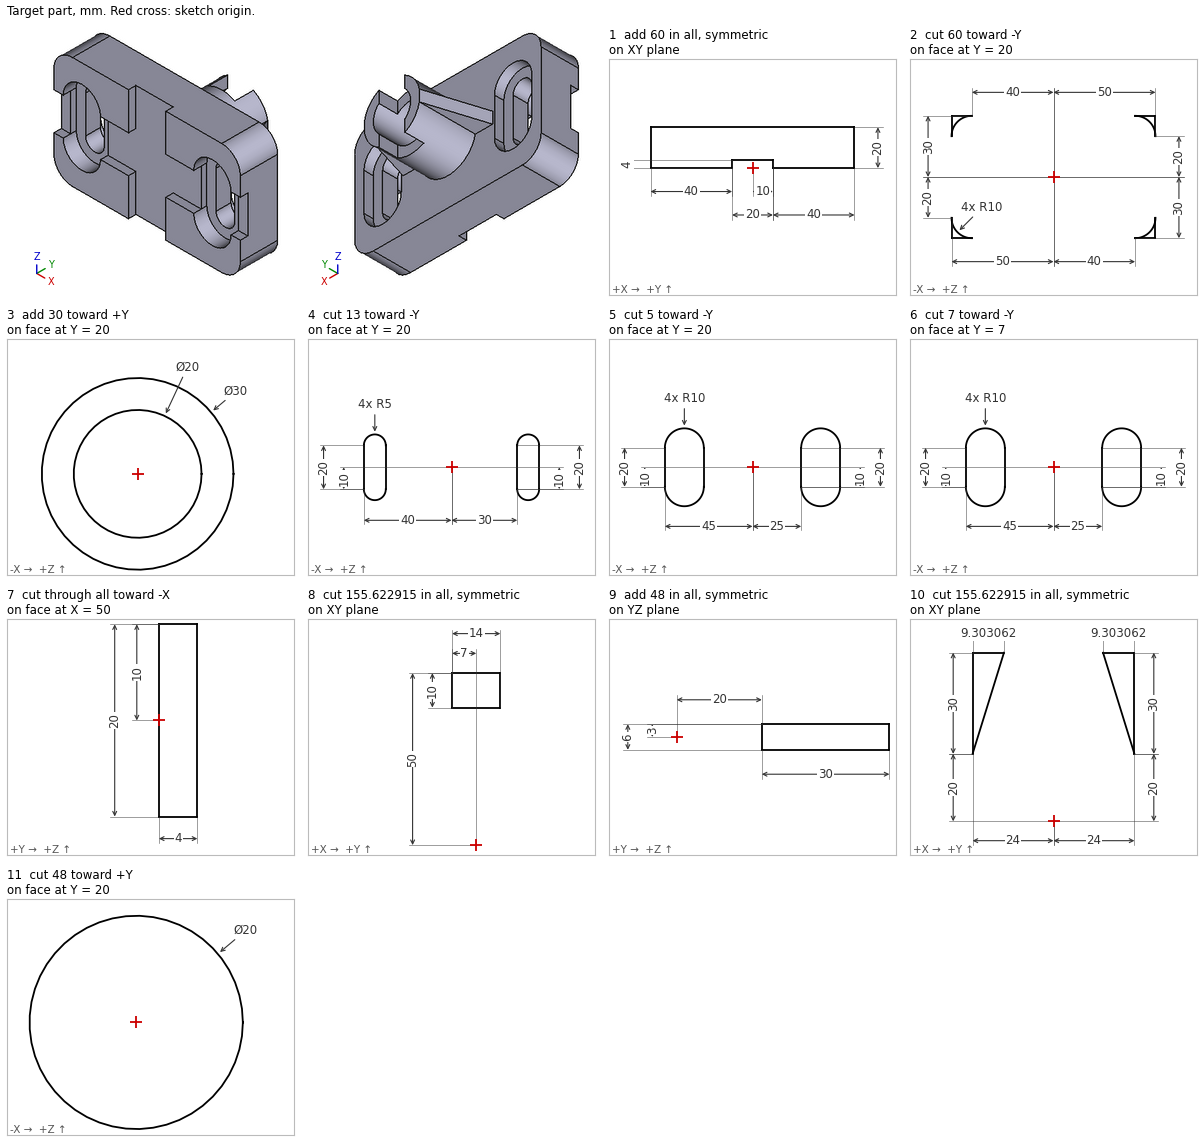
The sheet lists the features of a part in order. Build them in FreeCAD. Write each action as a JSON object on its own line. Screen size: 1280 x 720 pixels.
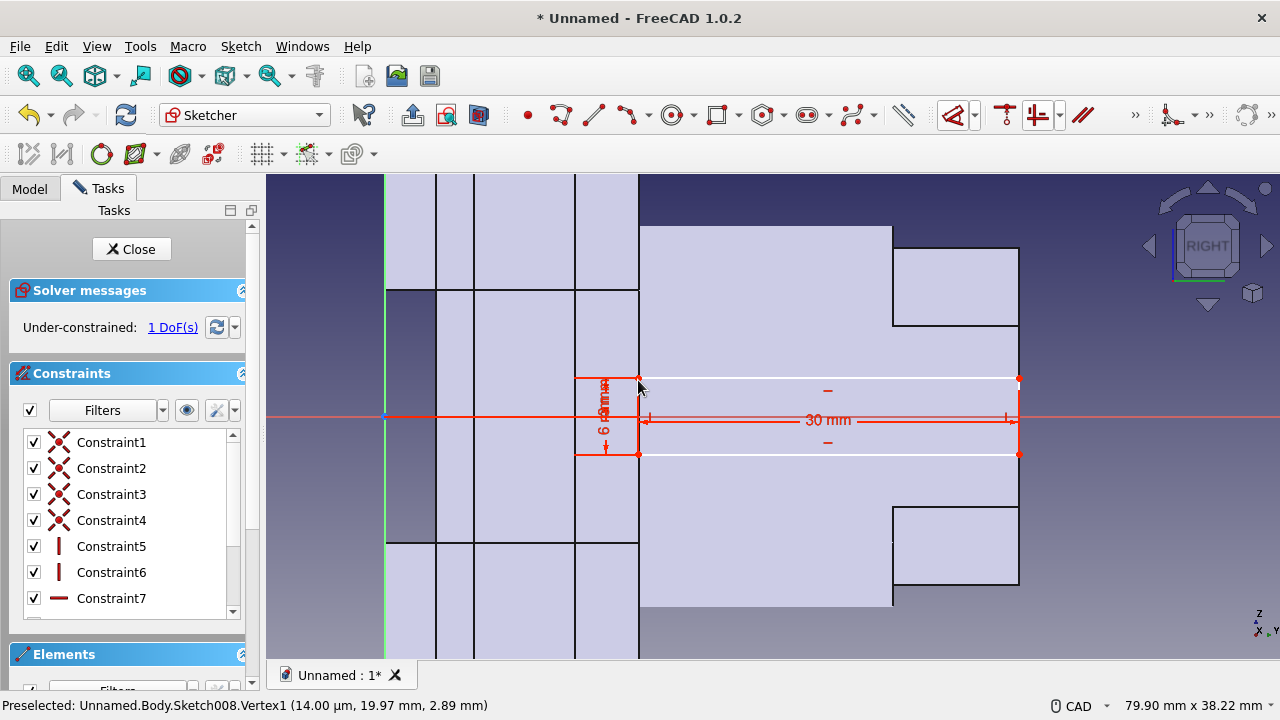
{"action": "left_click", "coordinate": [638, 378]}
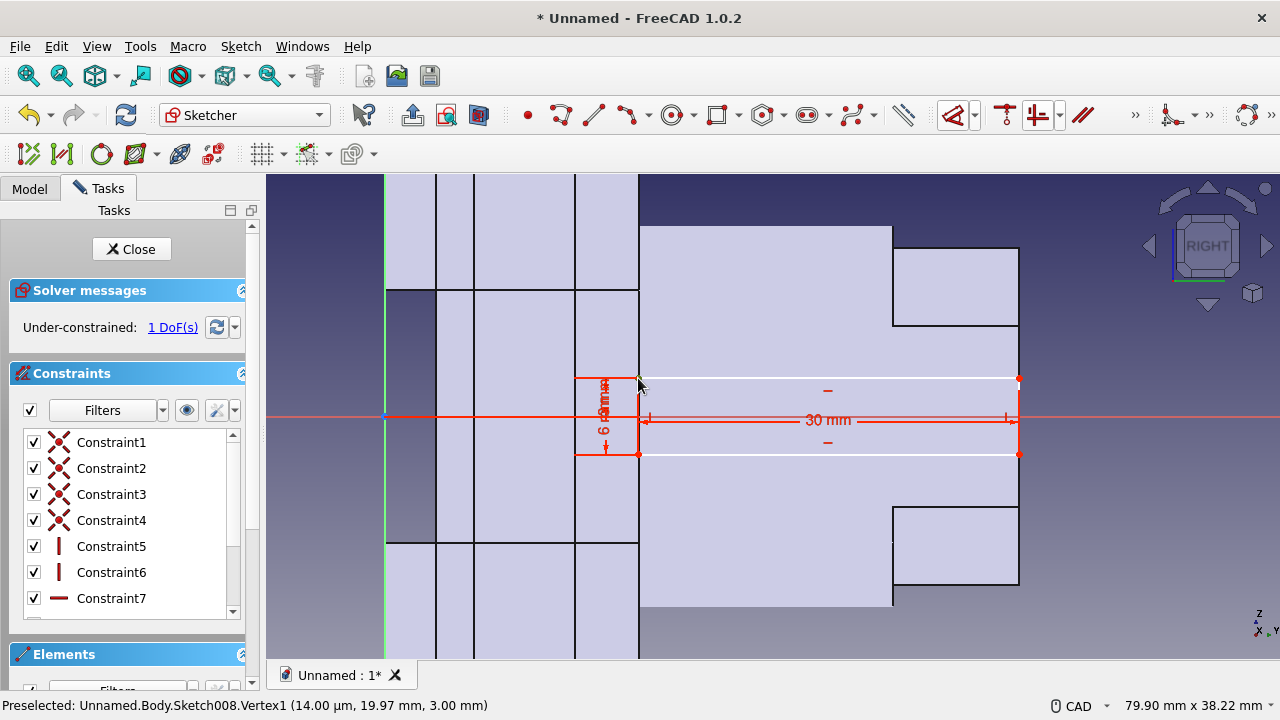
{"action": "key", "text": "l"}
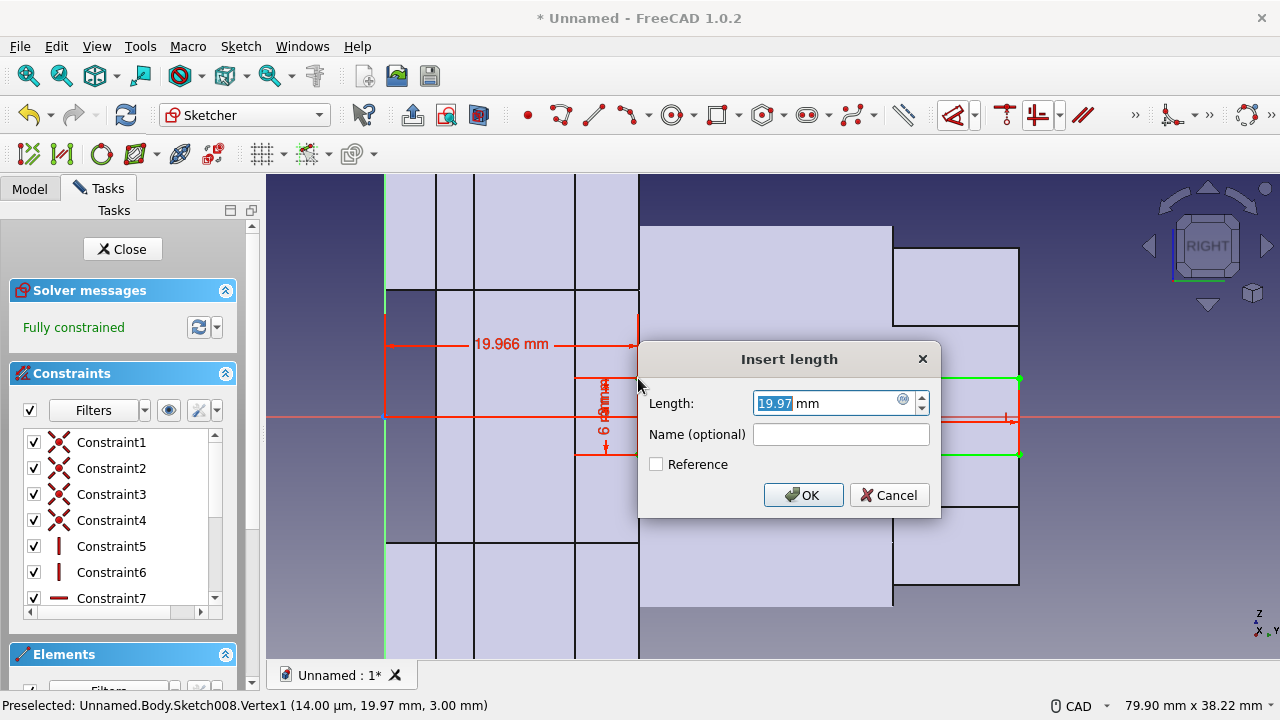
{"action": "type", "text": "20"}
{"action": "key", "text": "Return"}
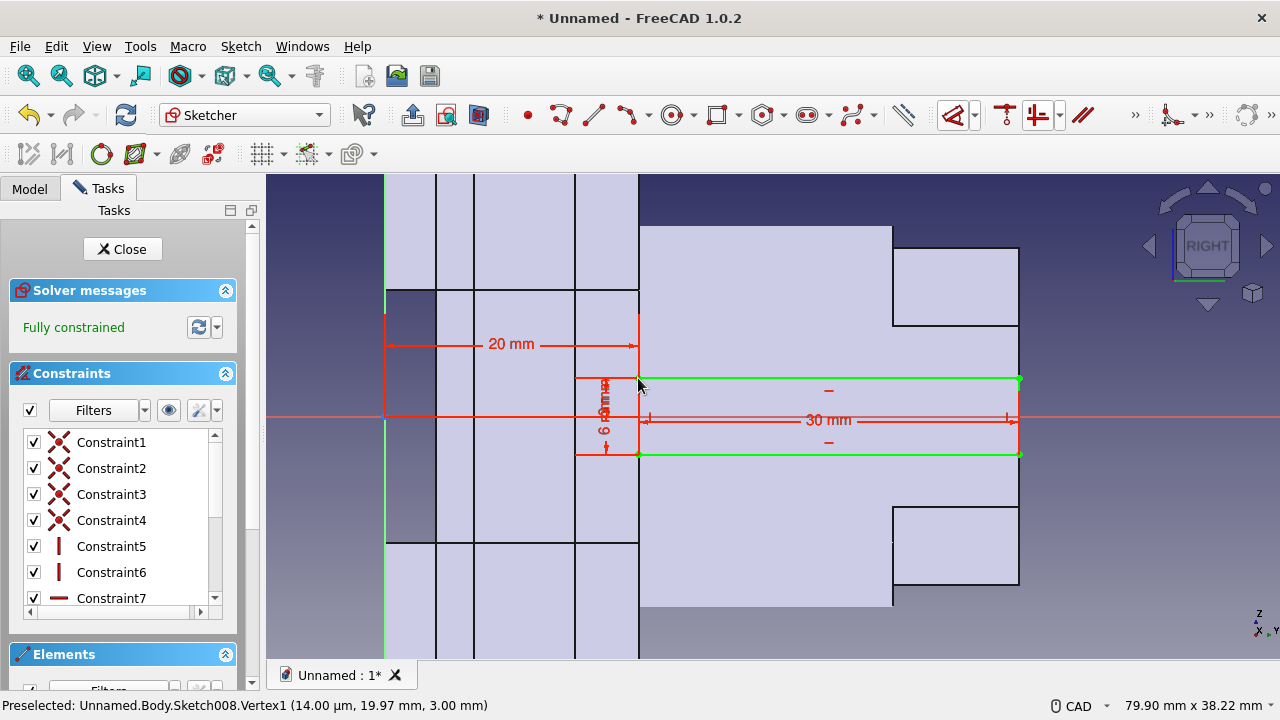
{"action": "left_click", "coordinate": [123, 249]}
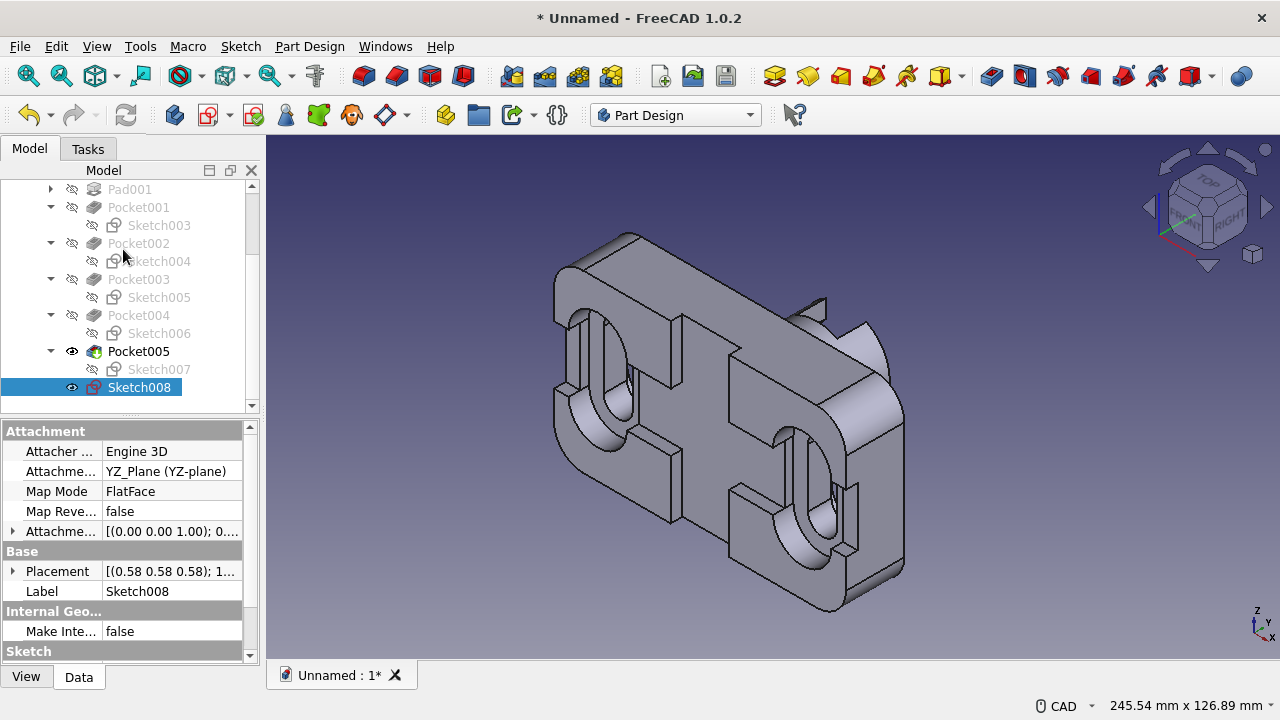
{"action": "left_click", "coordinate": [775, 76]}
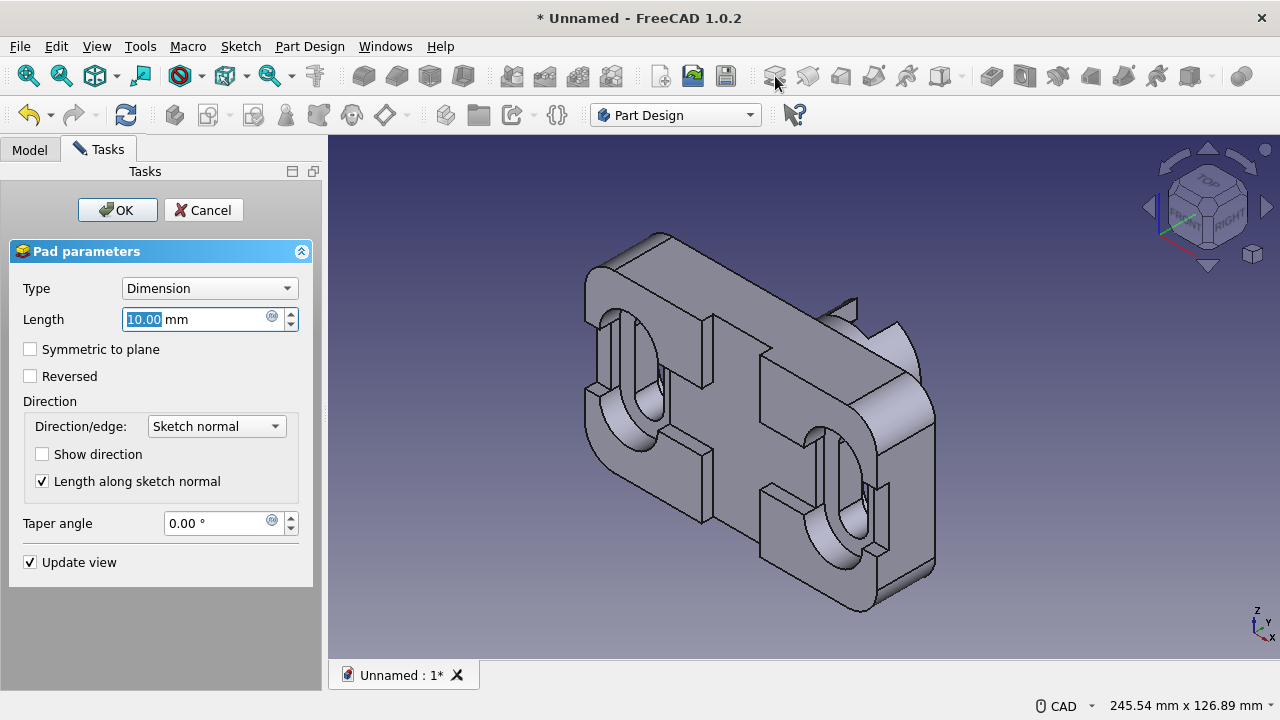
{"action": "type", "text": "48"}
{"action": "key", "text": "Tab"}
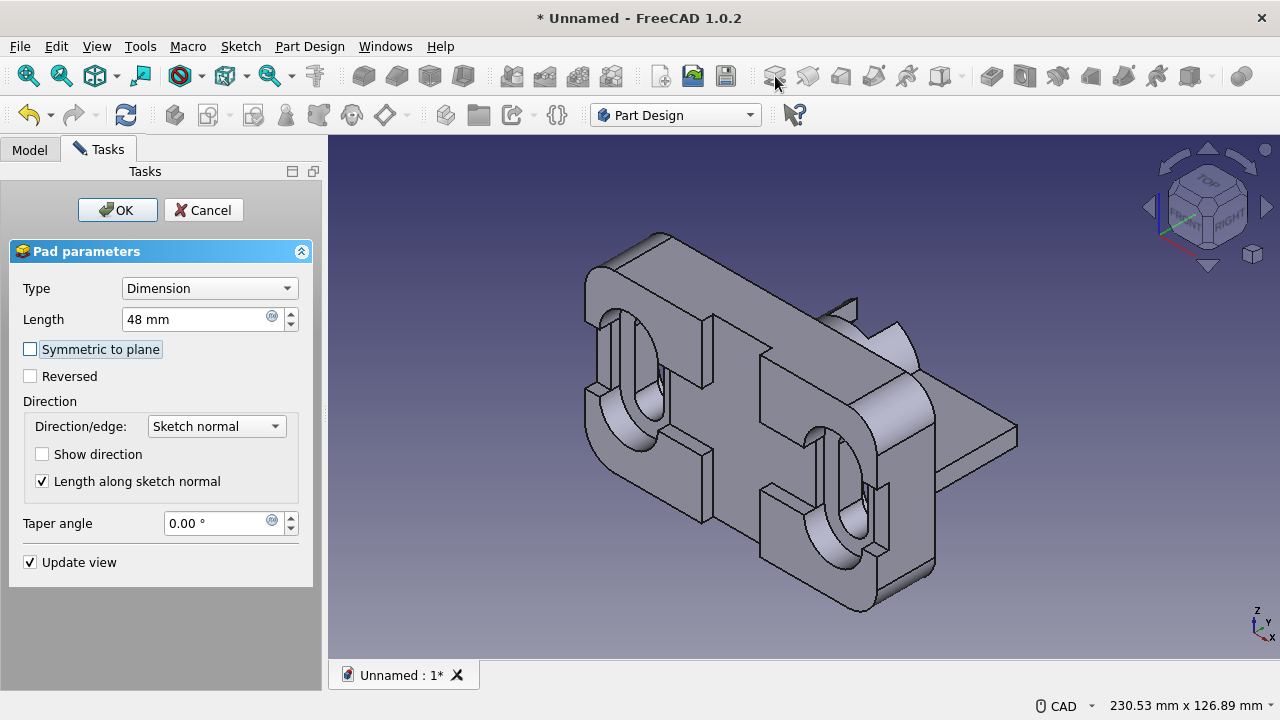
{"action": "left_click", "coordinate": [31, 349]}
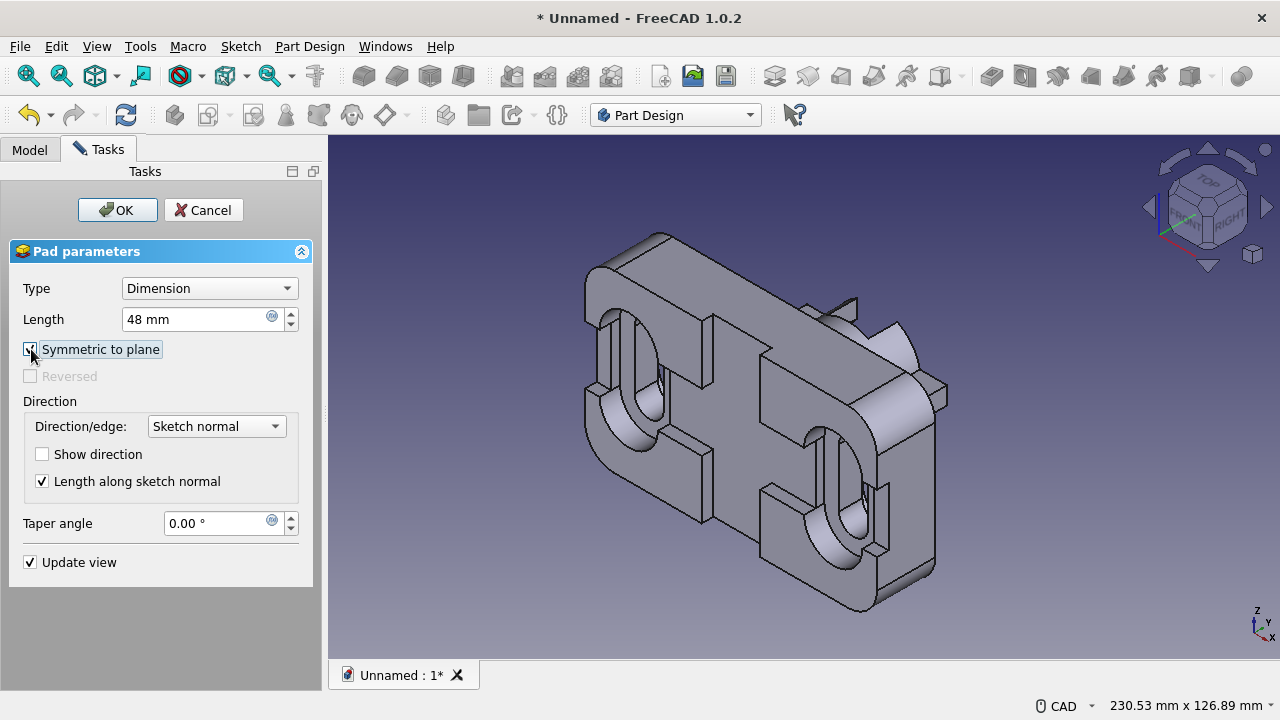
{"action": "left_click", "coordinate": [118, 210]}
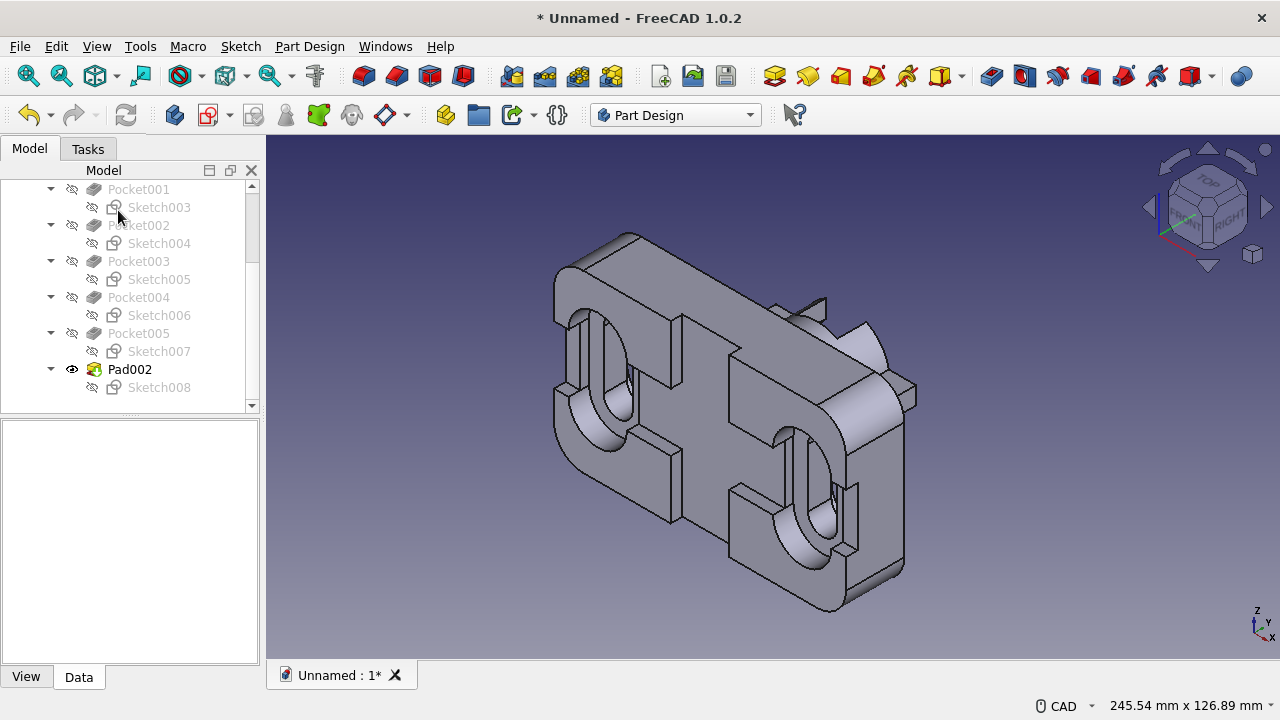
{"action": "left_click", "coordinate": [208, 116]}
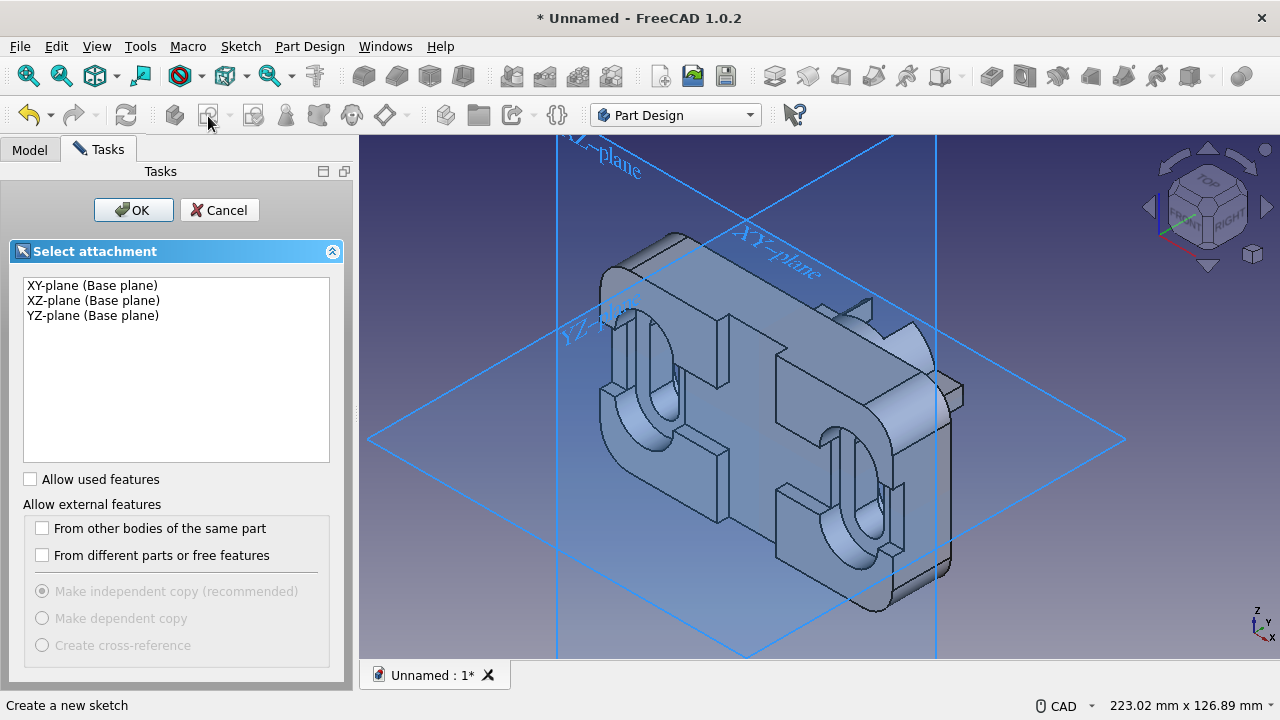
{"action": "left_click", "coordinate": [84, 286]}